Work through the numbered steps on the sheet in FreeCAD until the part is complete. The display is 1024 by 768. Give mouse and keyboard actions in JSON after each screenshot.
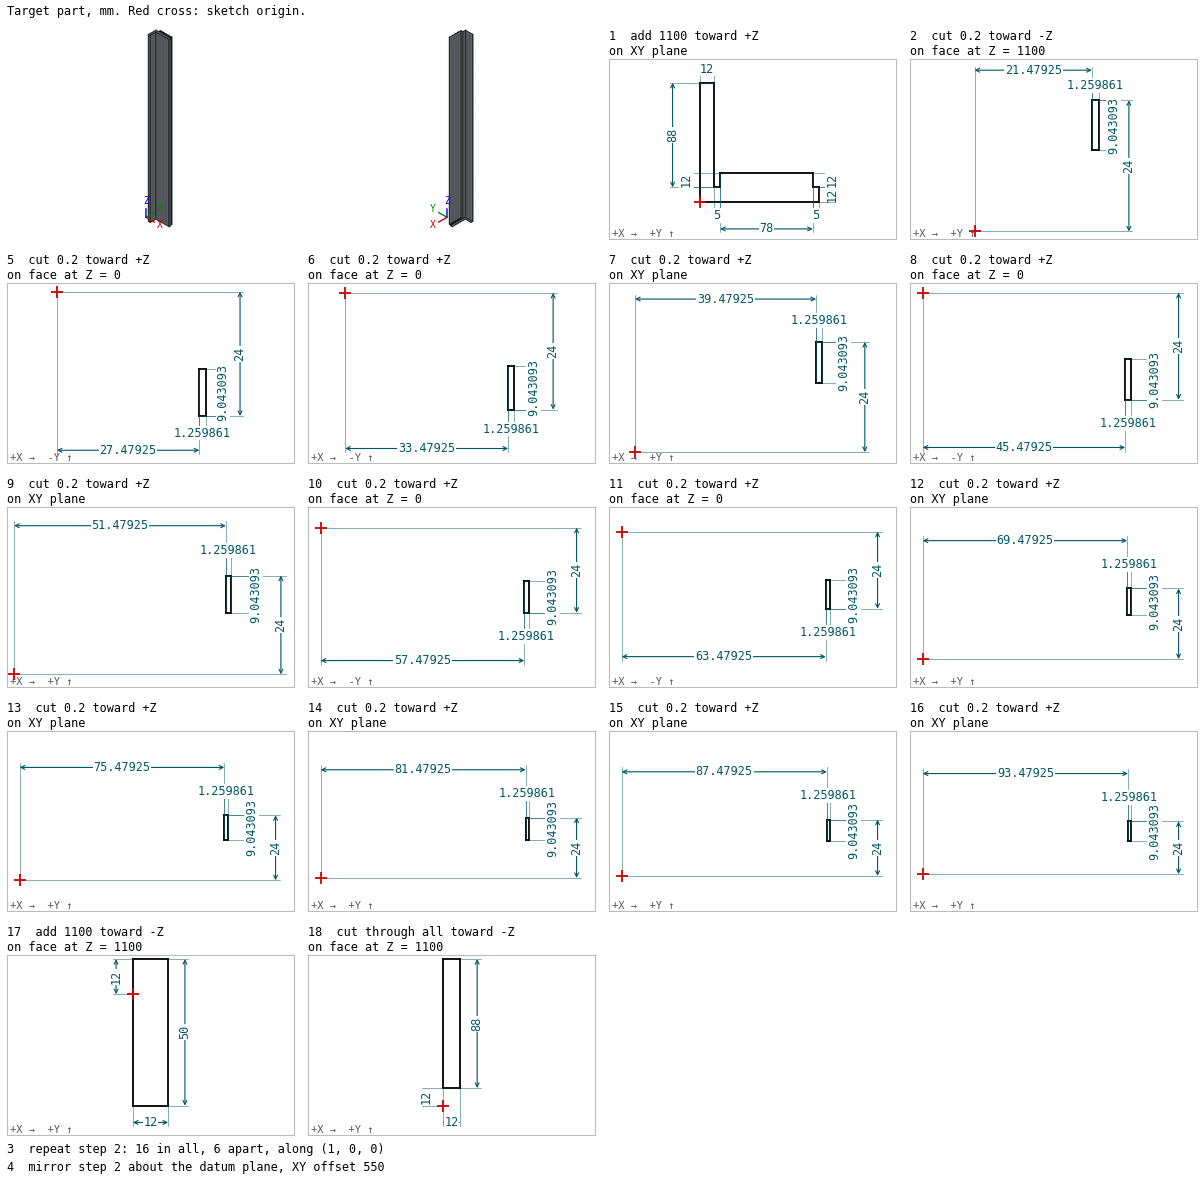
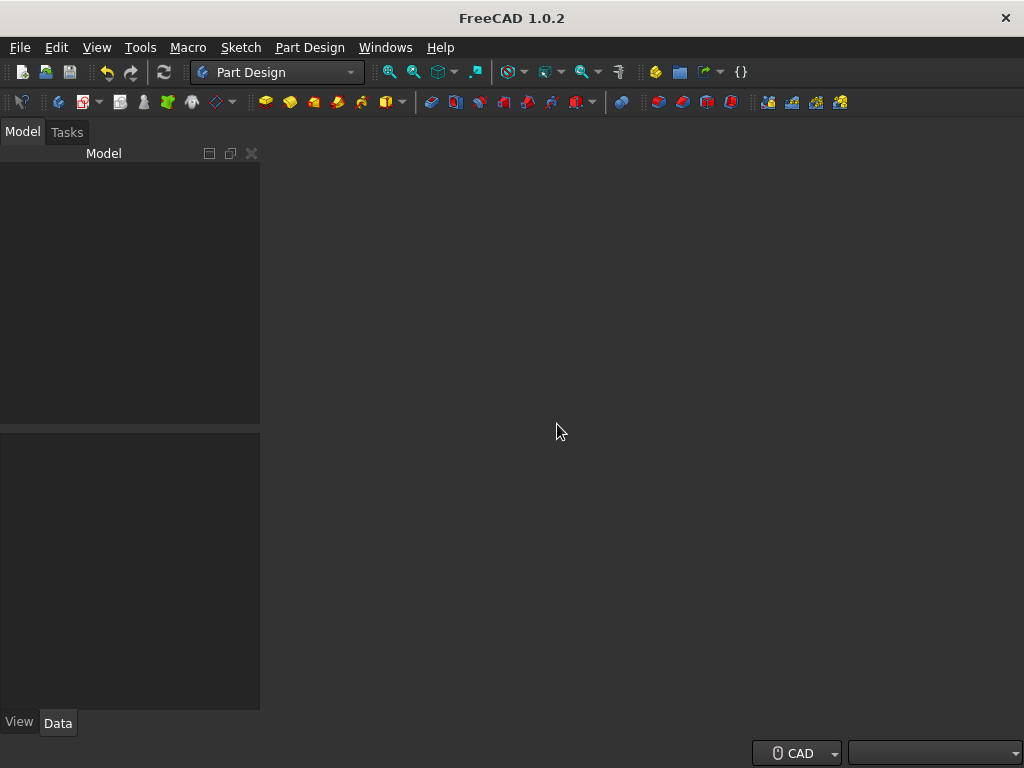
{"action": "left_click", "coordinate": [22, 72]}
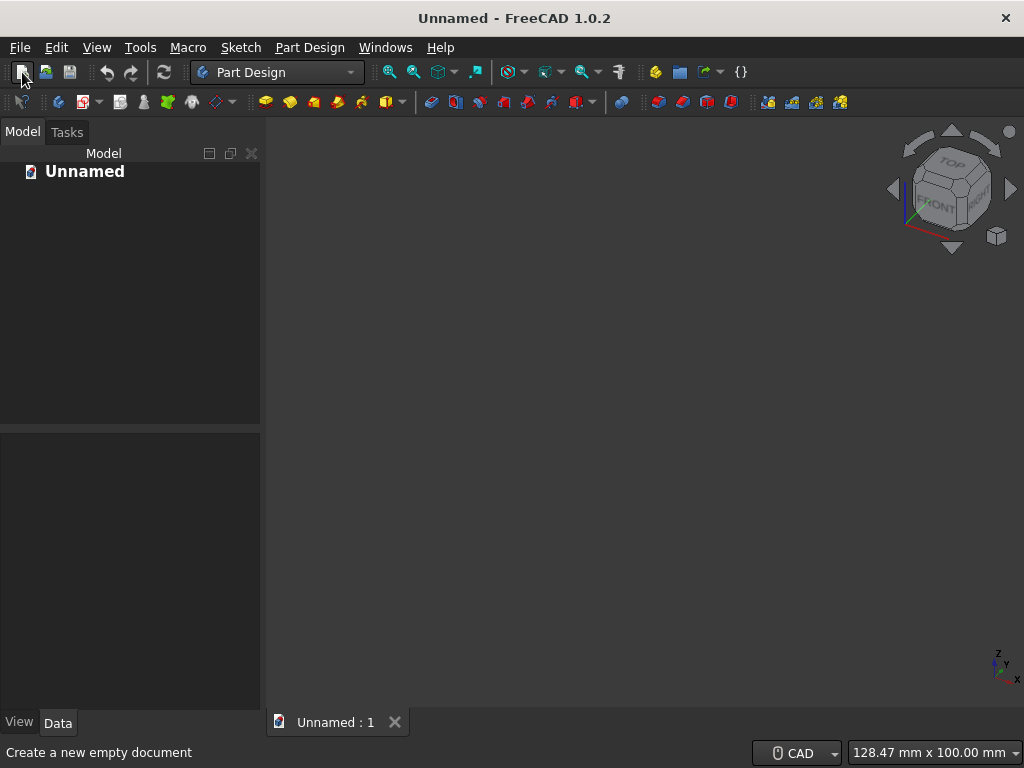
{"action": "left_click", "coordinate": [84, 102]}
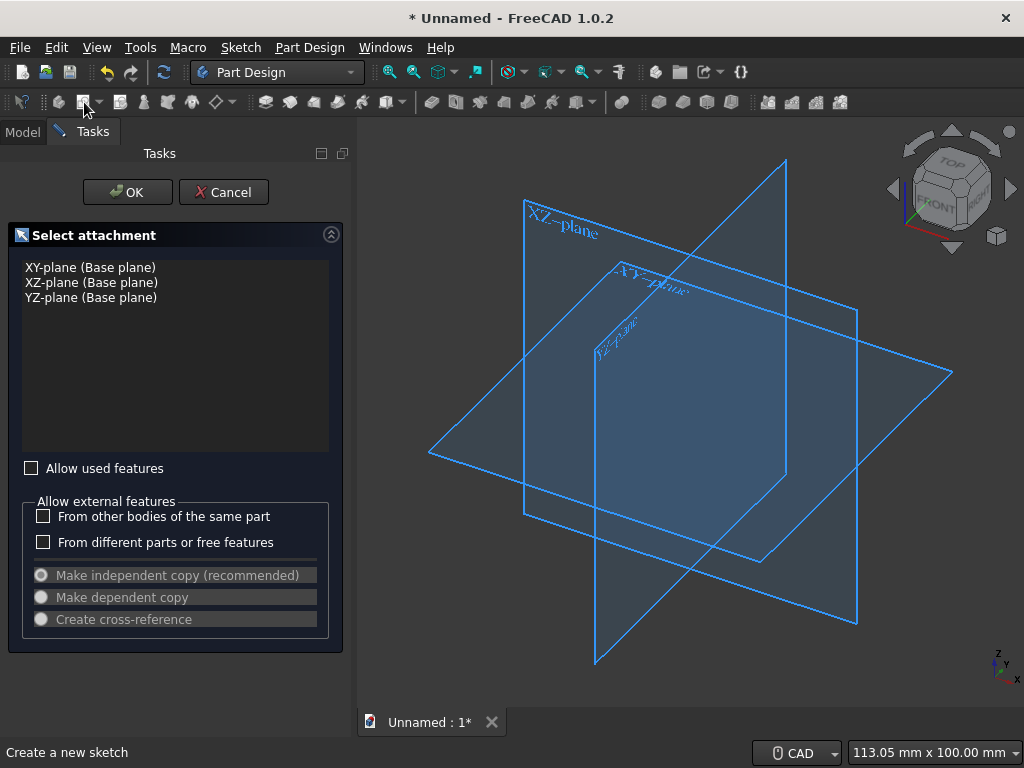
{"action": "left_click", "coordinate": [82, 268]}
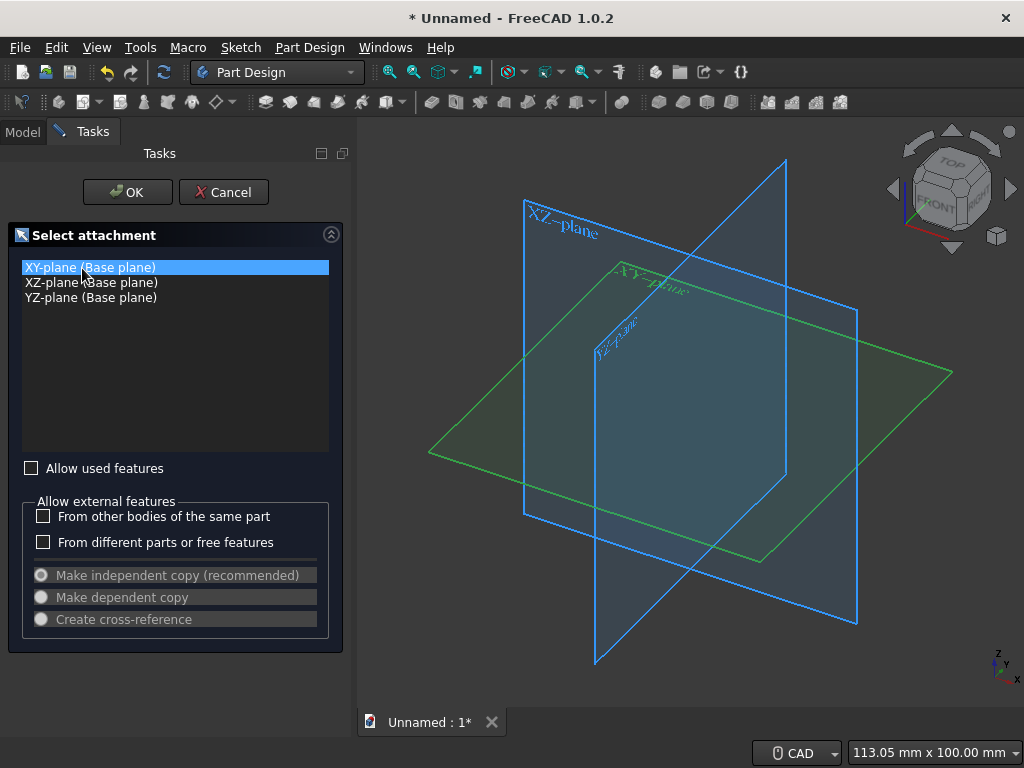
{"action": "left_click", "coordinate": [128, 192]}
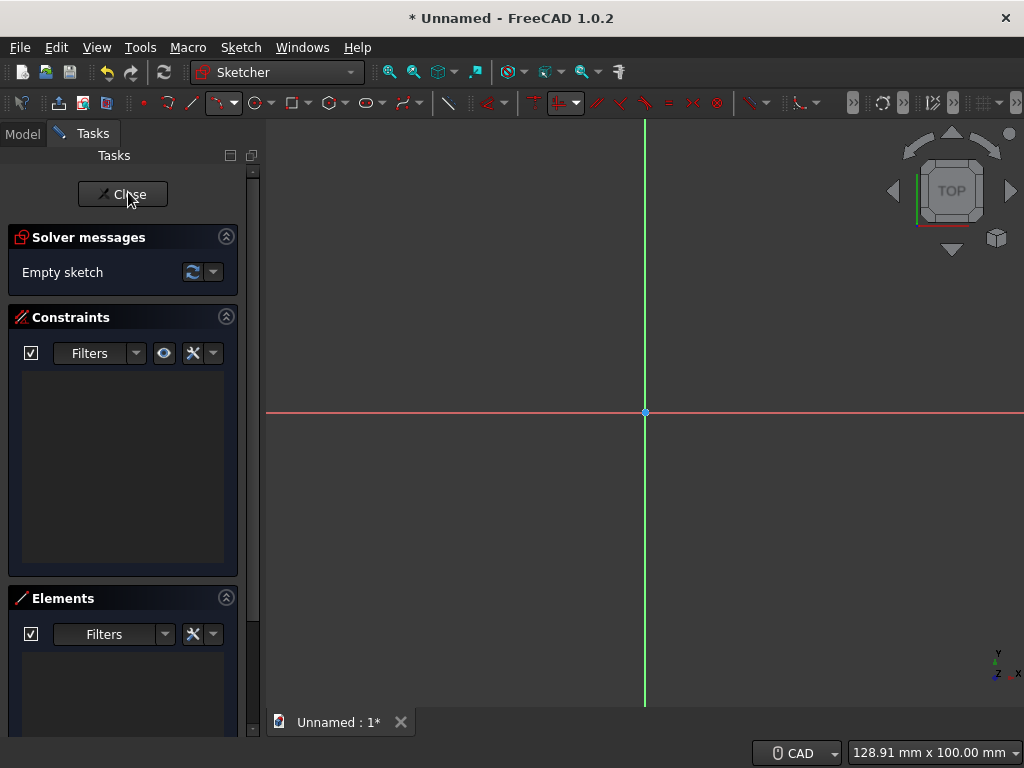
{"action": "scroll", "coordinate": [294, 679], "scroll_direction": "down", "scroll_amount": 3}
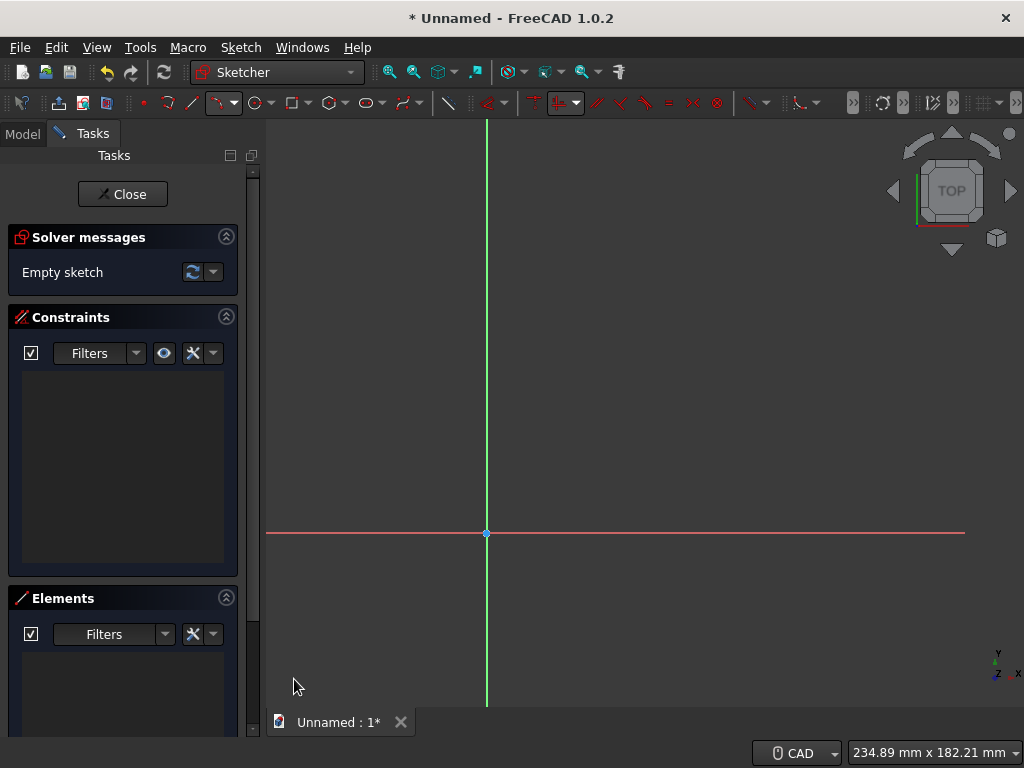
{"action": "left_click", "coordinate": [168, 104]}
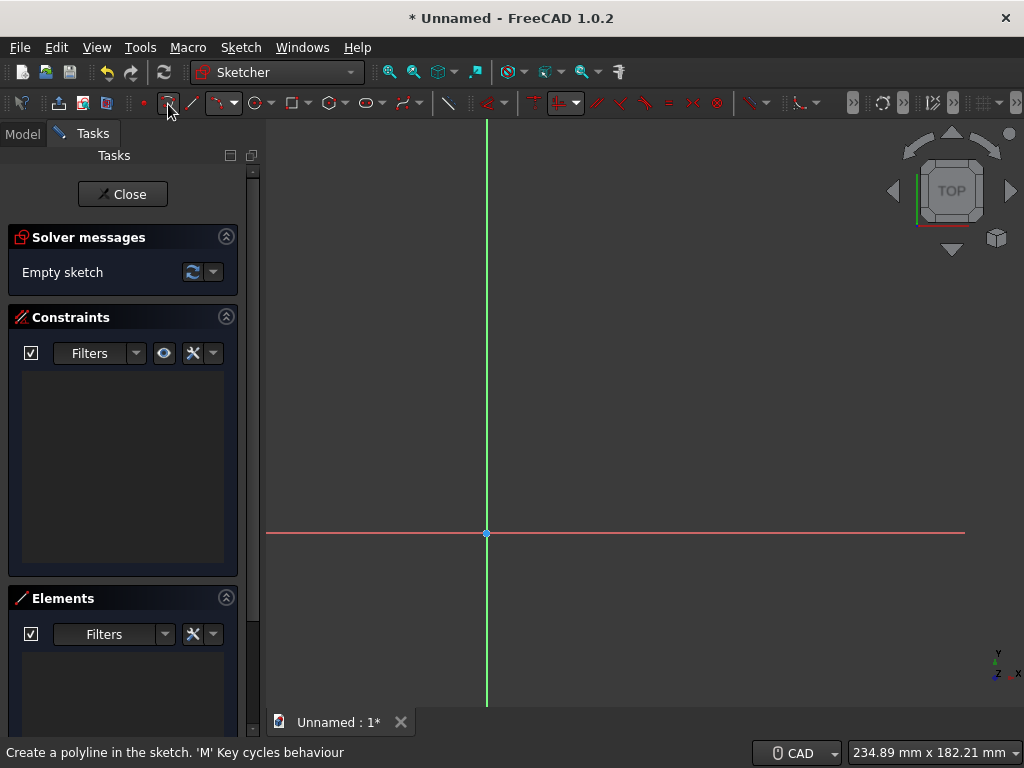
{"action": "left_click", "coordinate": [487, 533]}
{"action": "left_click", "coordinate": [809, 524]}
{"action": "left_click", "coordinate": [809, 495]}
{"action": "left_click", "coordinate": [793, 495]}
{"action": "left_click", "coordinate": [793, 456]}
{"action": "left_click", "coordinate": [542, 456]}
{"action": "left_click", "coordinate": [542, 495]}
{"action": "left_click", "coordinate": [525, 495]}
{"action": "left_click", "coordinate": [525, 211]}
{"action": "left_click", "coordinate": [496, 211]}
{"action": "left_click", "coordinate": [487, 533]}
{"action": "key", "text": "Escape"}
{"action": "key", "text": "Escape"}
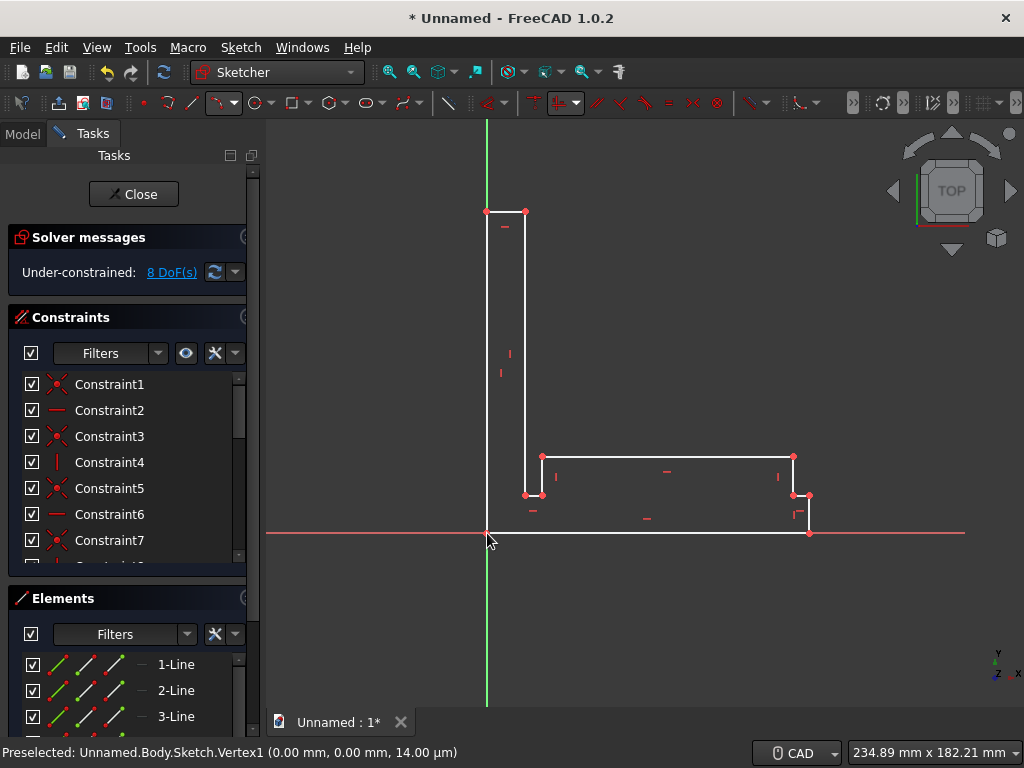
{"action": "scroll", "coordinate": [801, 496], "scroll_direction": "up", "scroll_amount": 5}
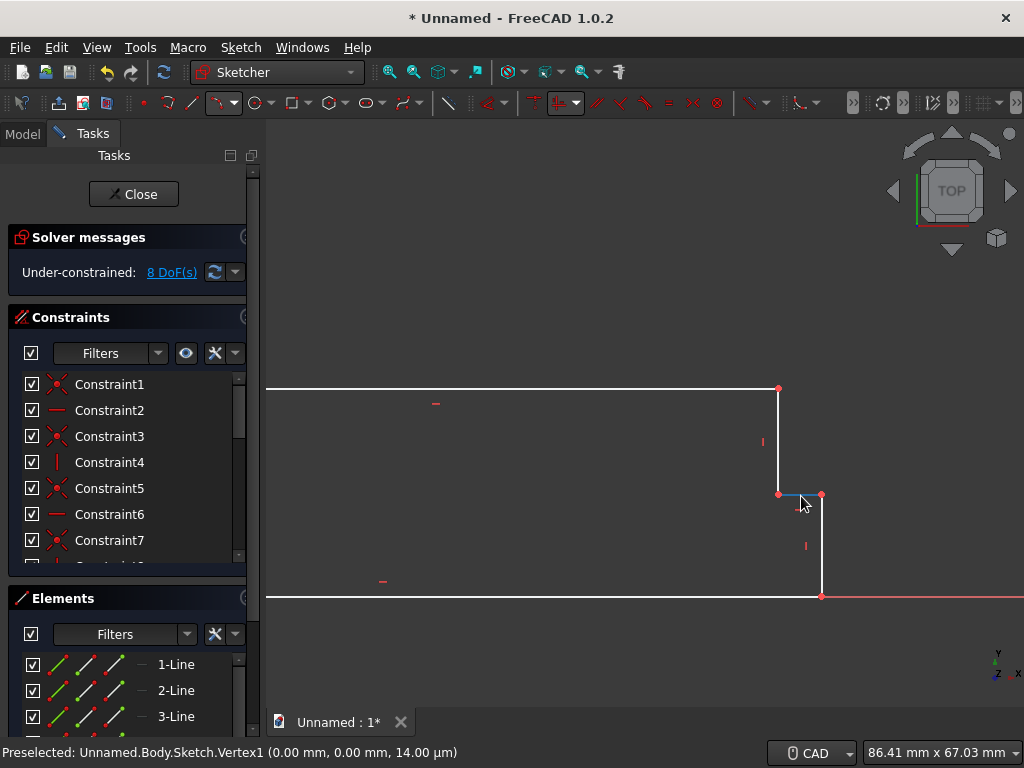
{"action": "left_click", "coordinate": [800, 495]}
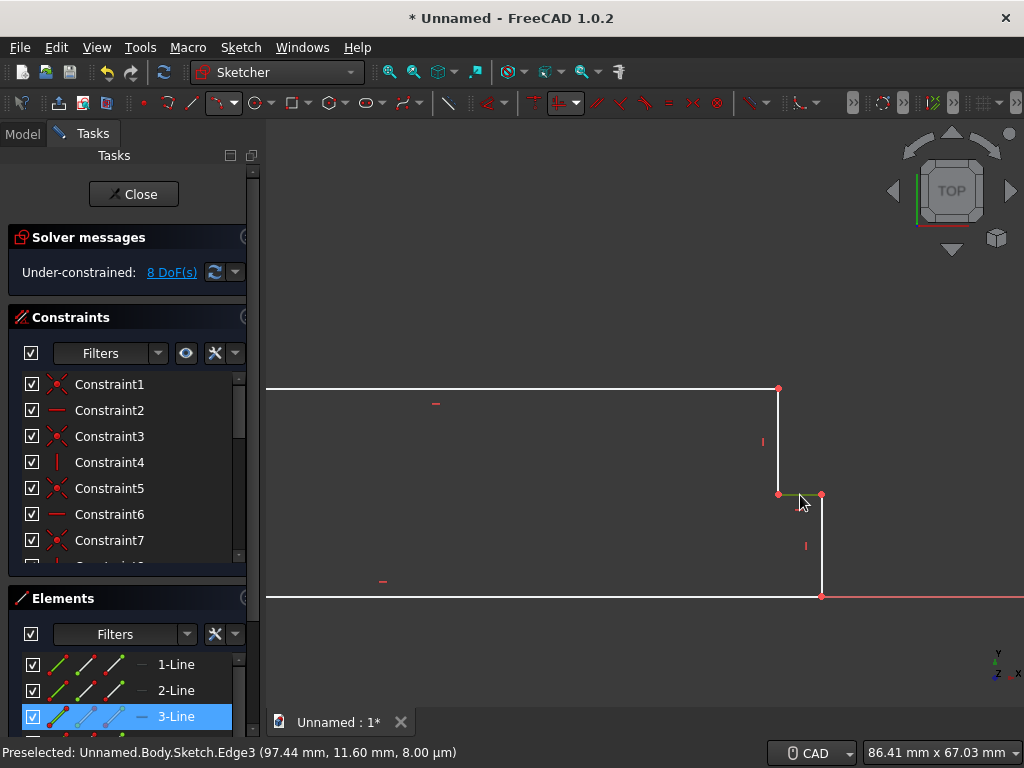
{"action": "left_click", "coordinate": [506, 104]}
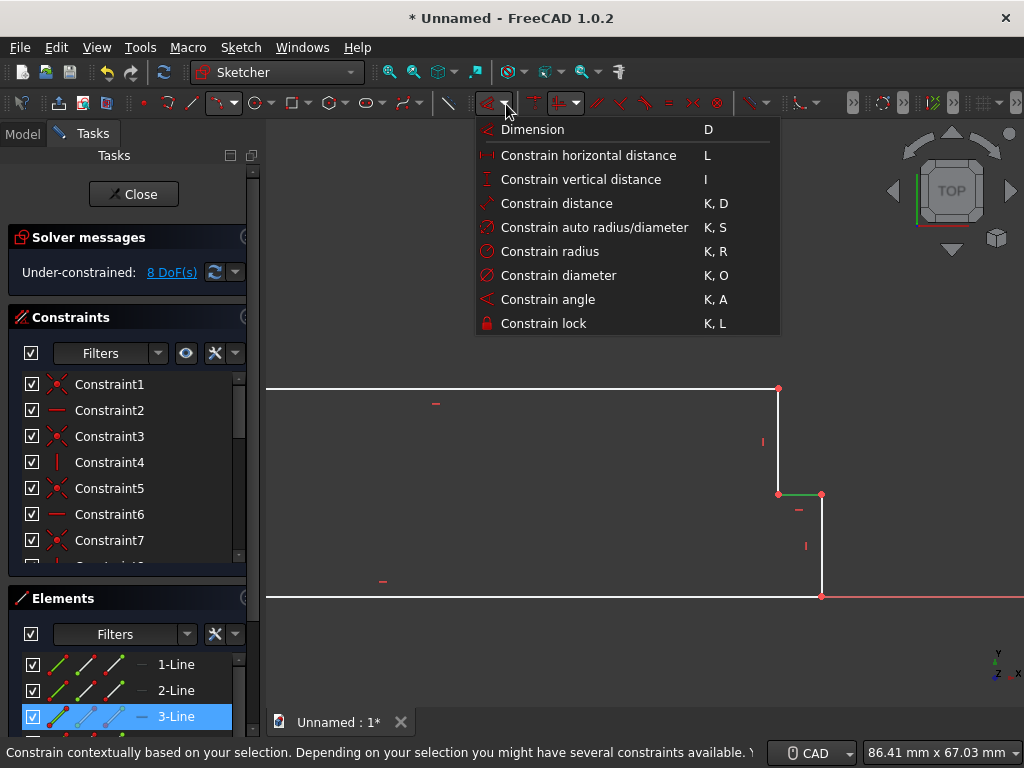
{"action": "left_click", "coordinate": [628, 155]}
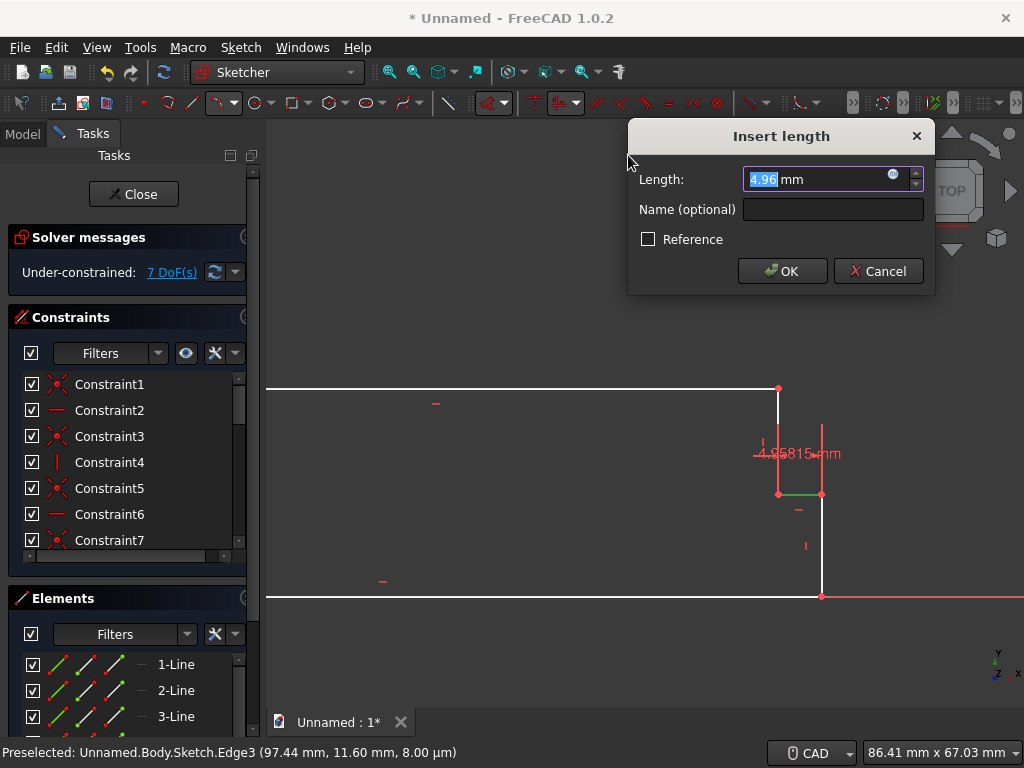
{"action": "type", "text": "5"}
{"action": "key", "text": "Return"}